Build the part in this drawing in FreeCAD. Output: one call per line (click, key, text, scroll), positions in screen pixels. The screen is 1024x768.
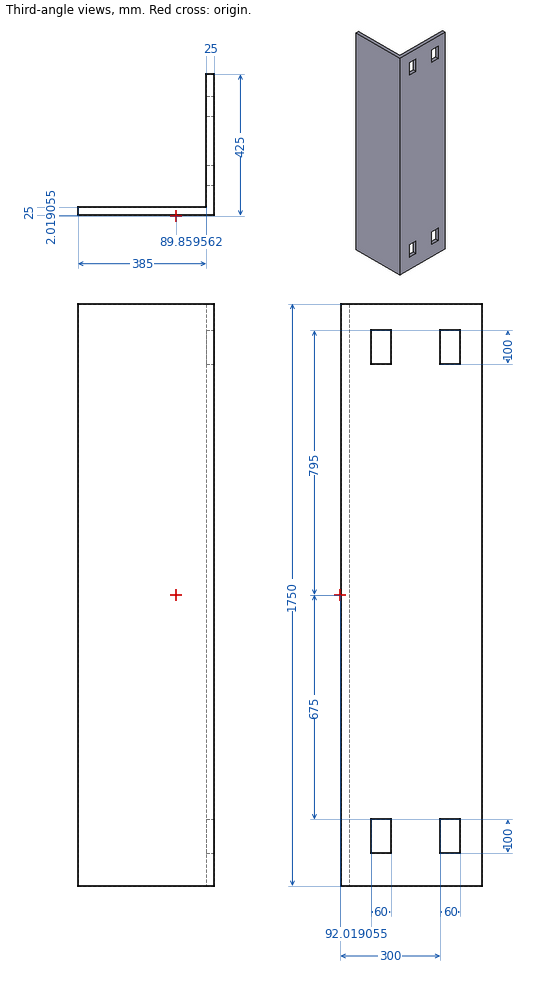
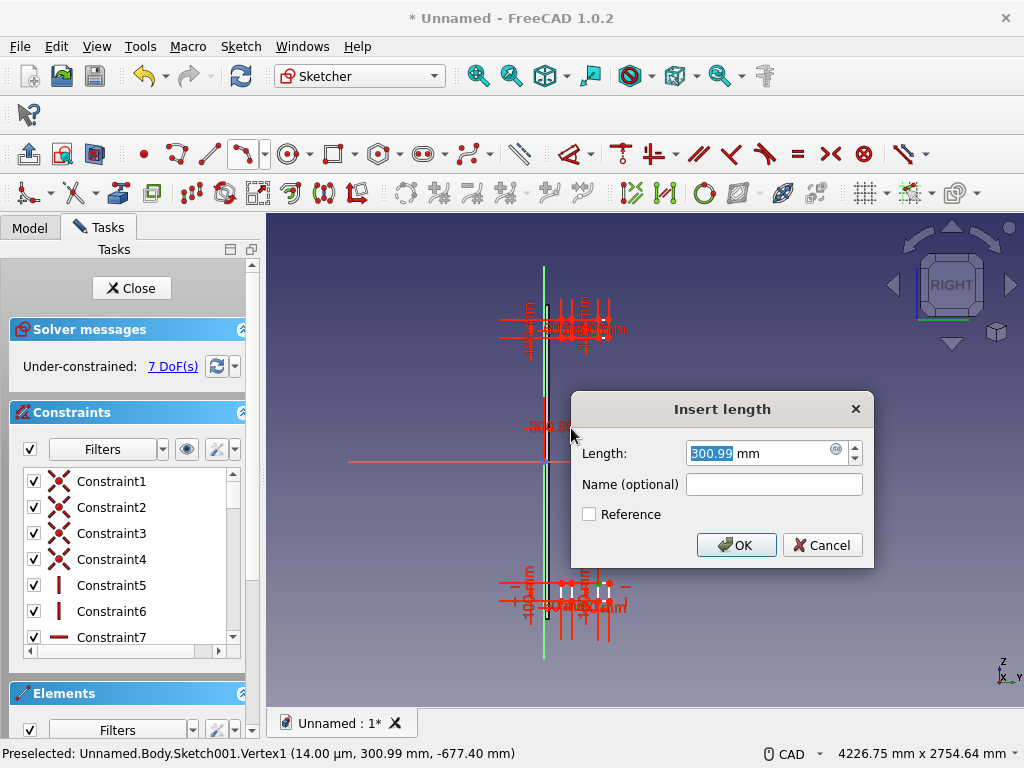
text(300)
key(Return)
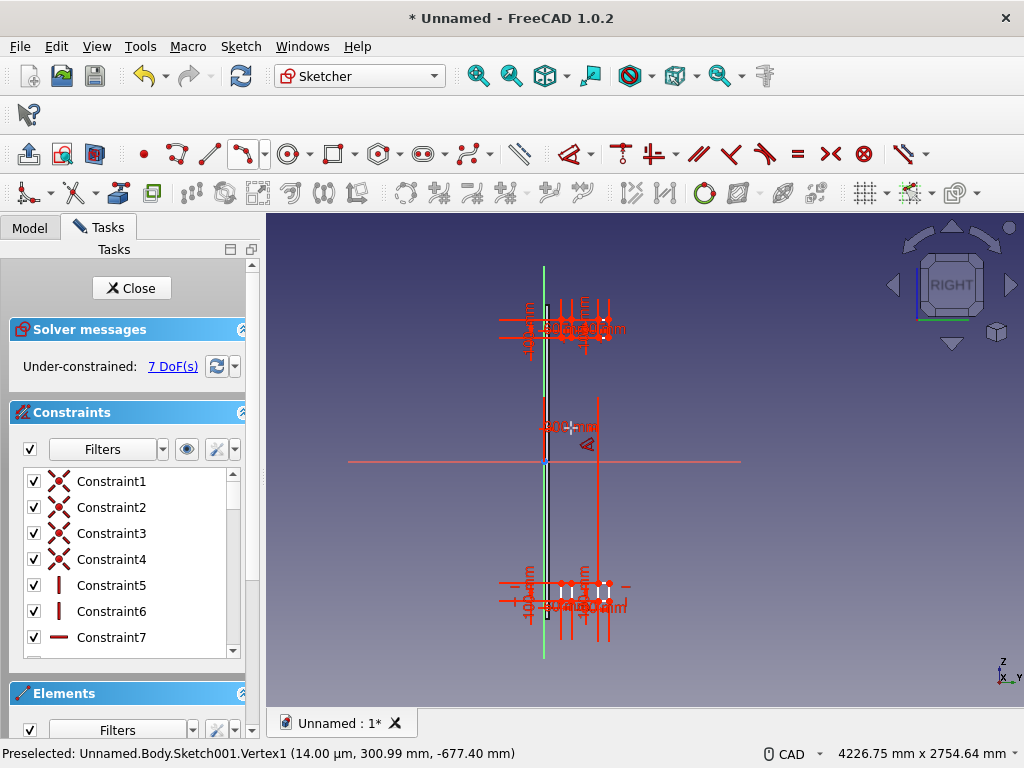
click(598, 583)
click(510, 523)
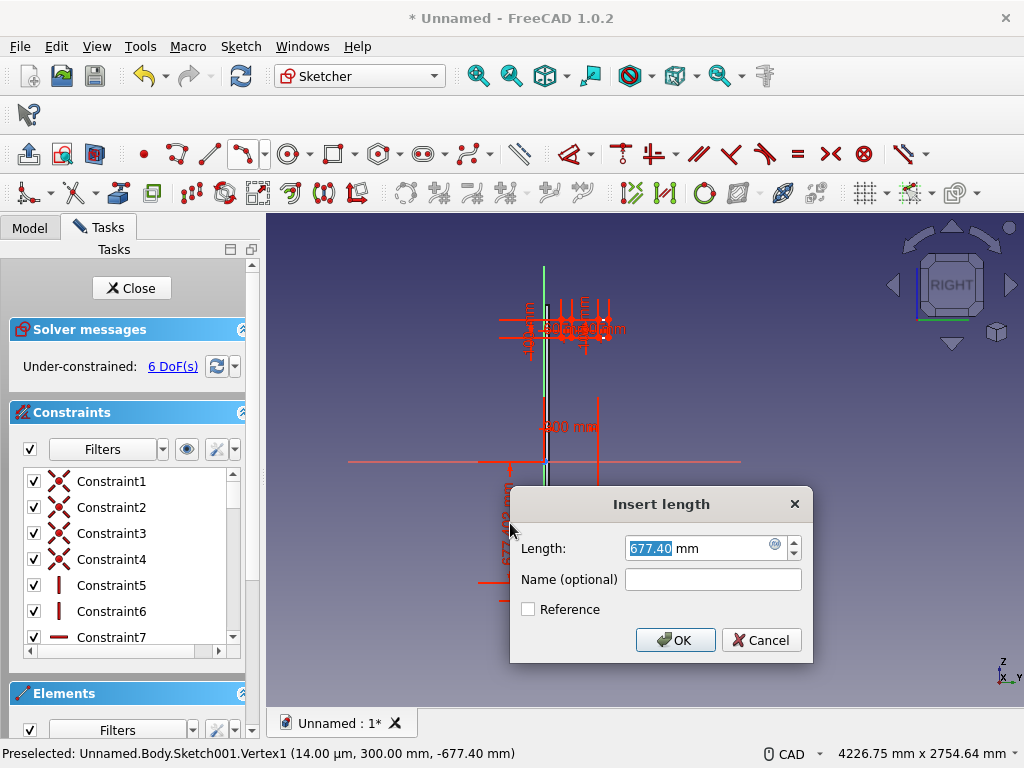
text(675)
key(Return)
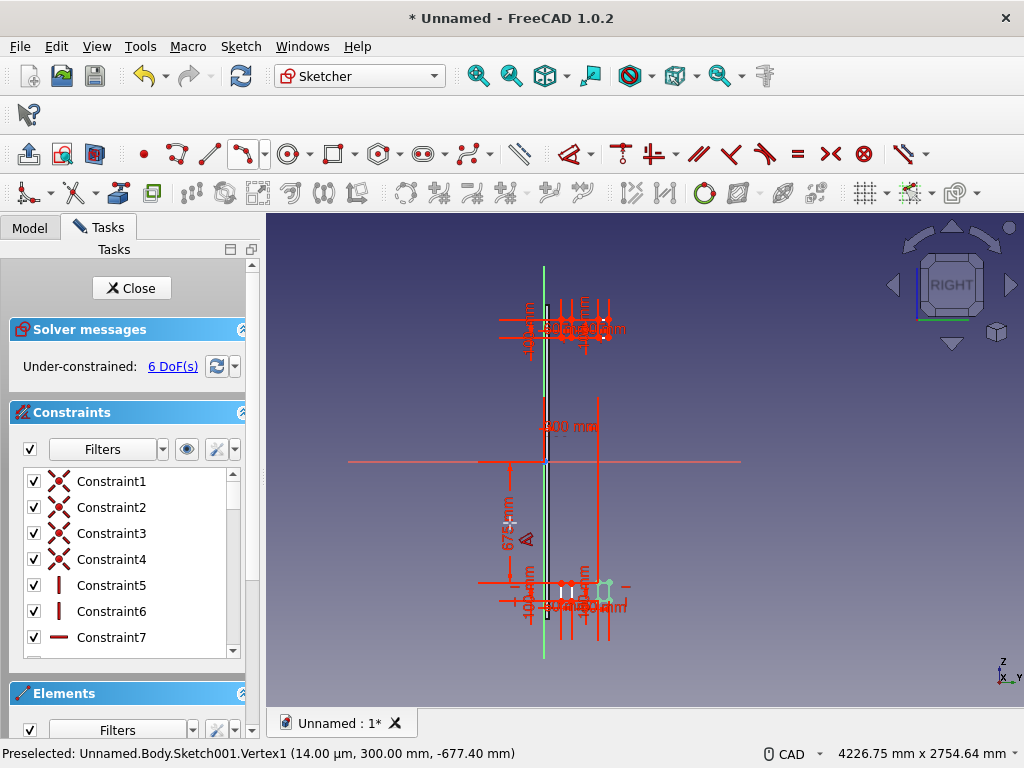
click(598, 320)
click(571, 286)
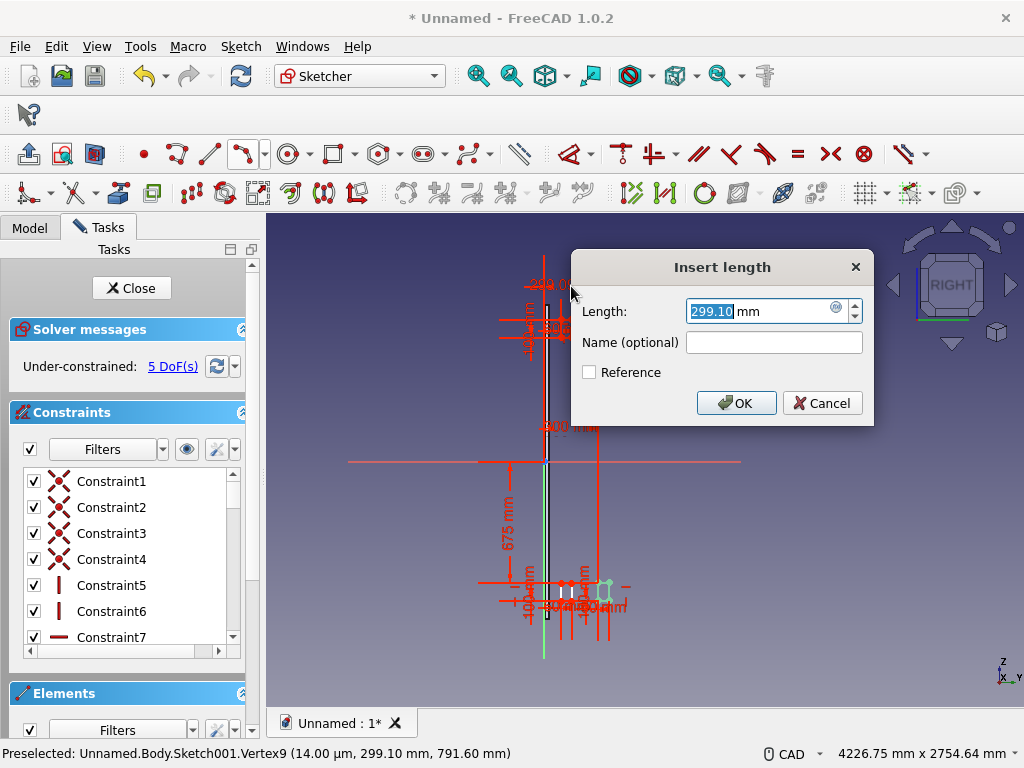
text(300)
key(Return)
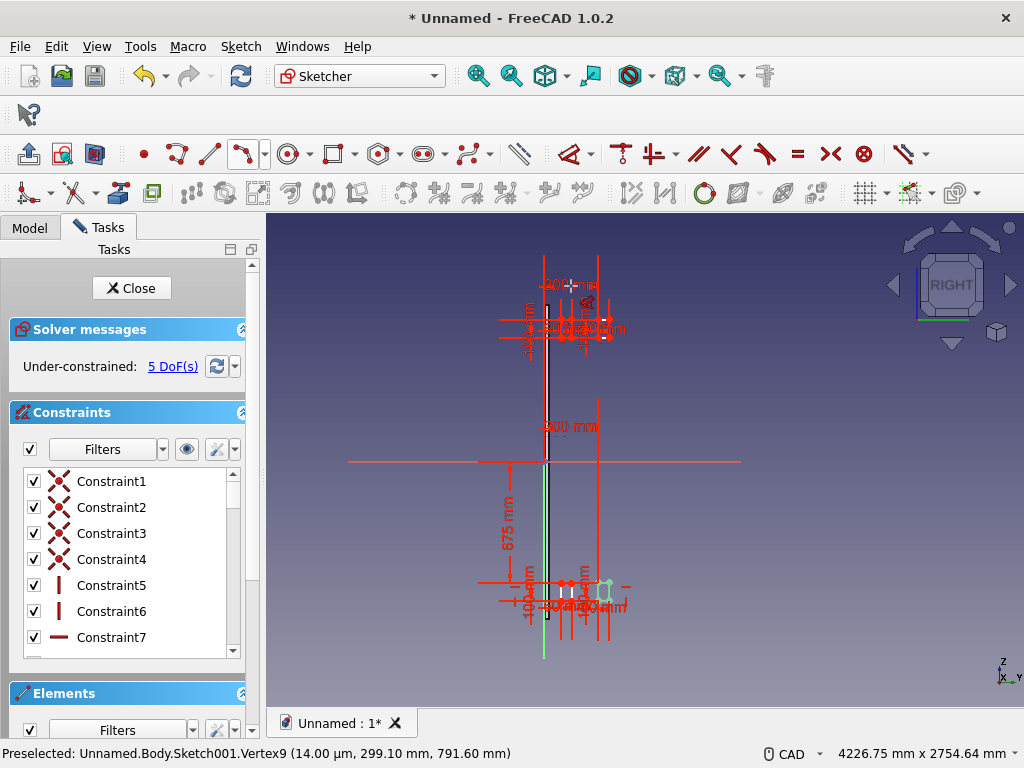
click(598, 320)
click(510, 391)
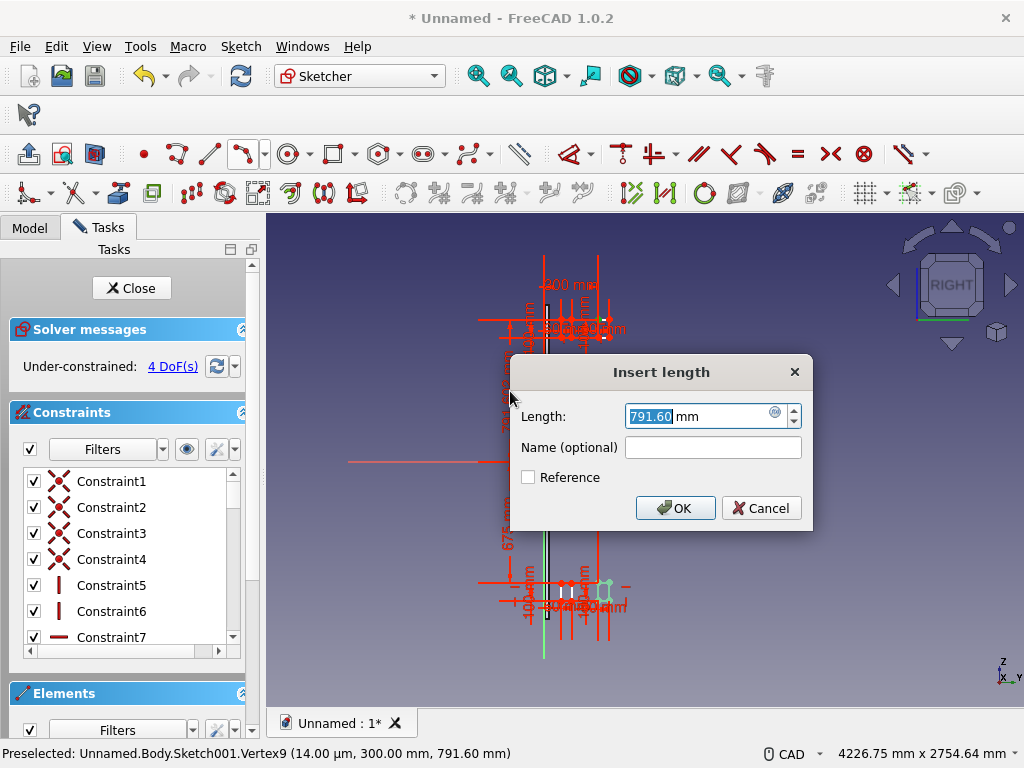
text(795)
key(Return)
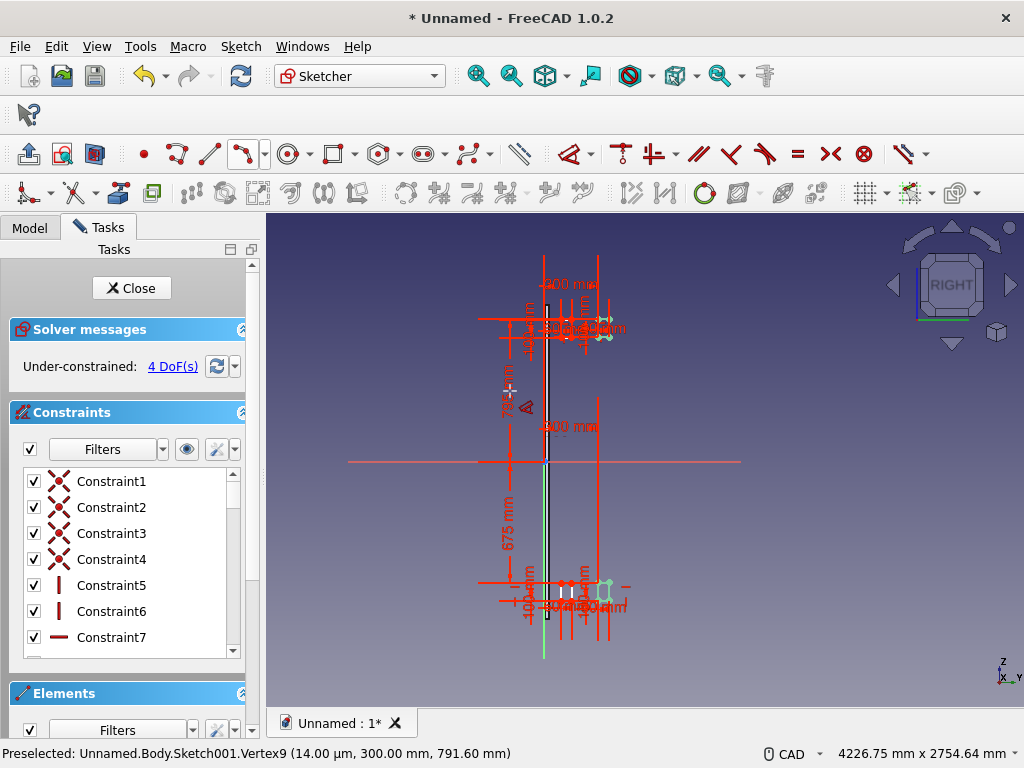
click(561, 583)
click(510, 495)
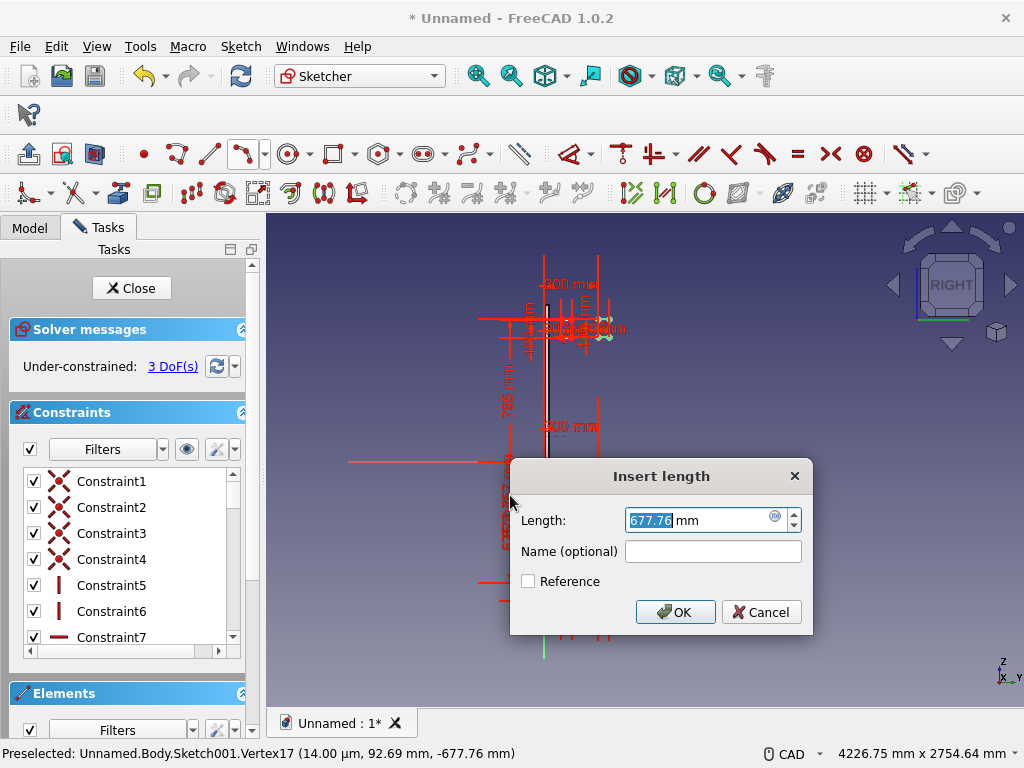
text(675)
key(Return)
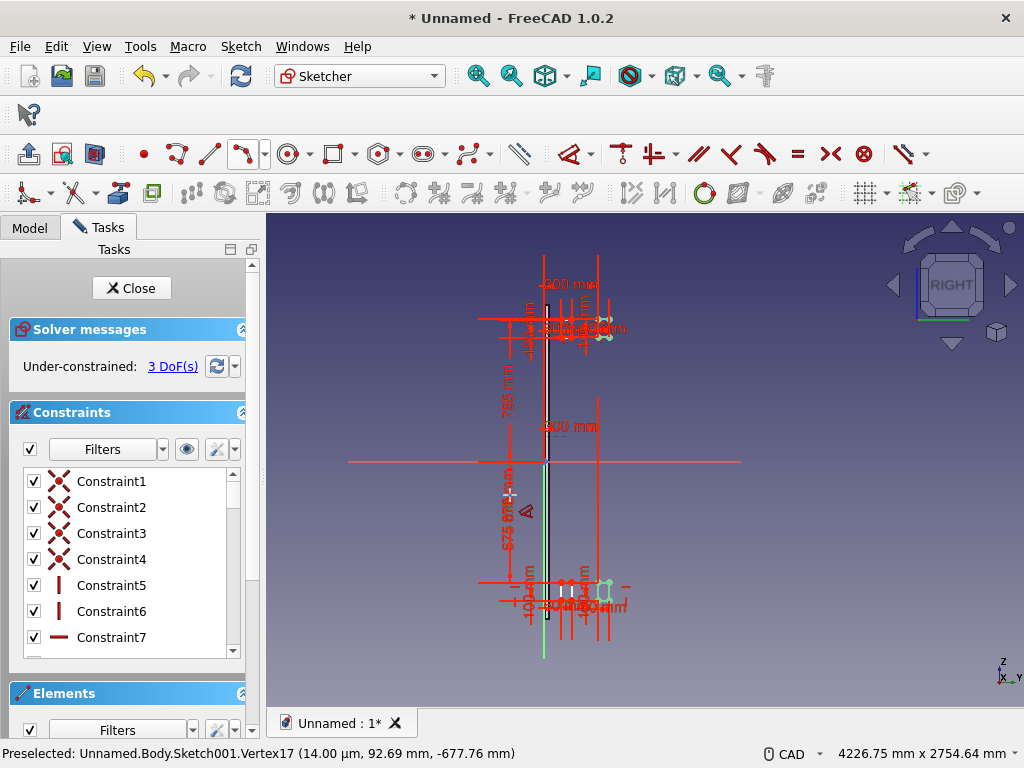
click(561, 320)
click(510, 358)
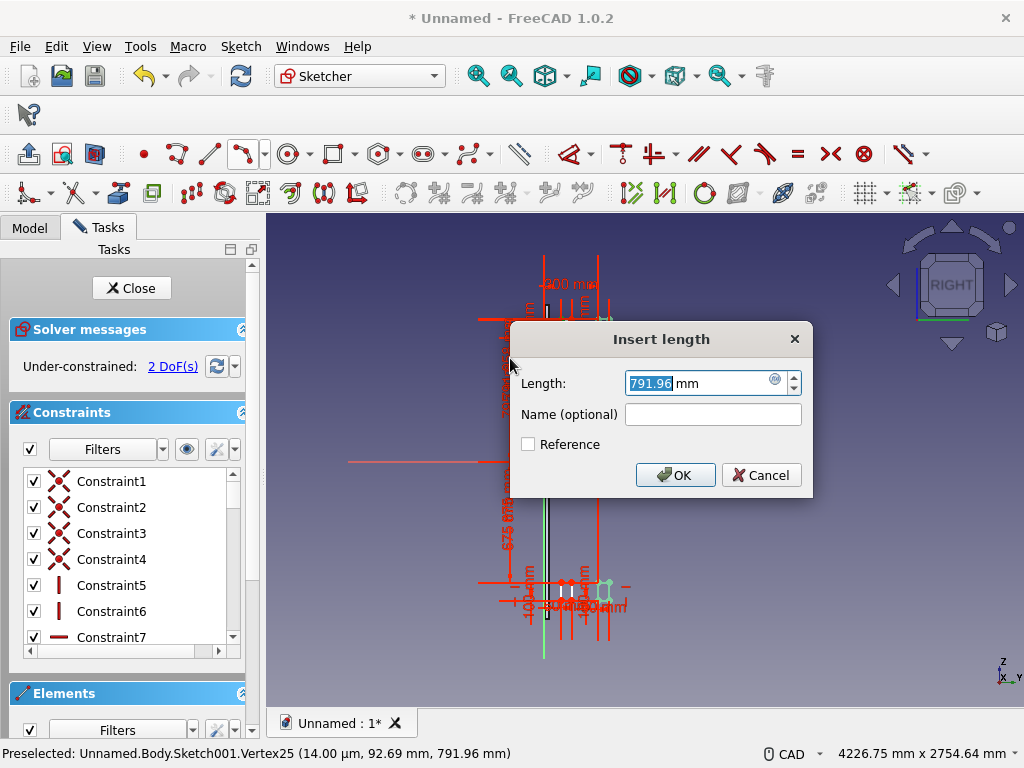
text(795)
key(Return)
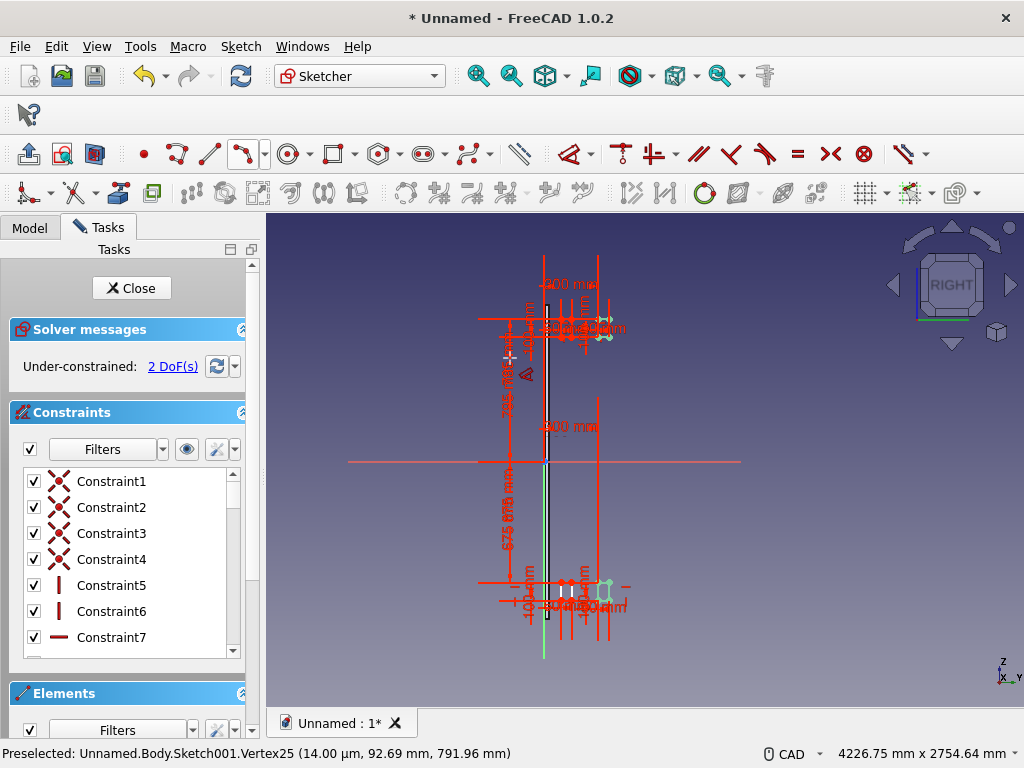
scroll(561, 583, up, 5)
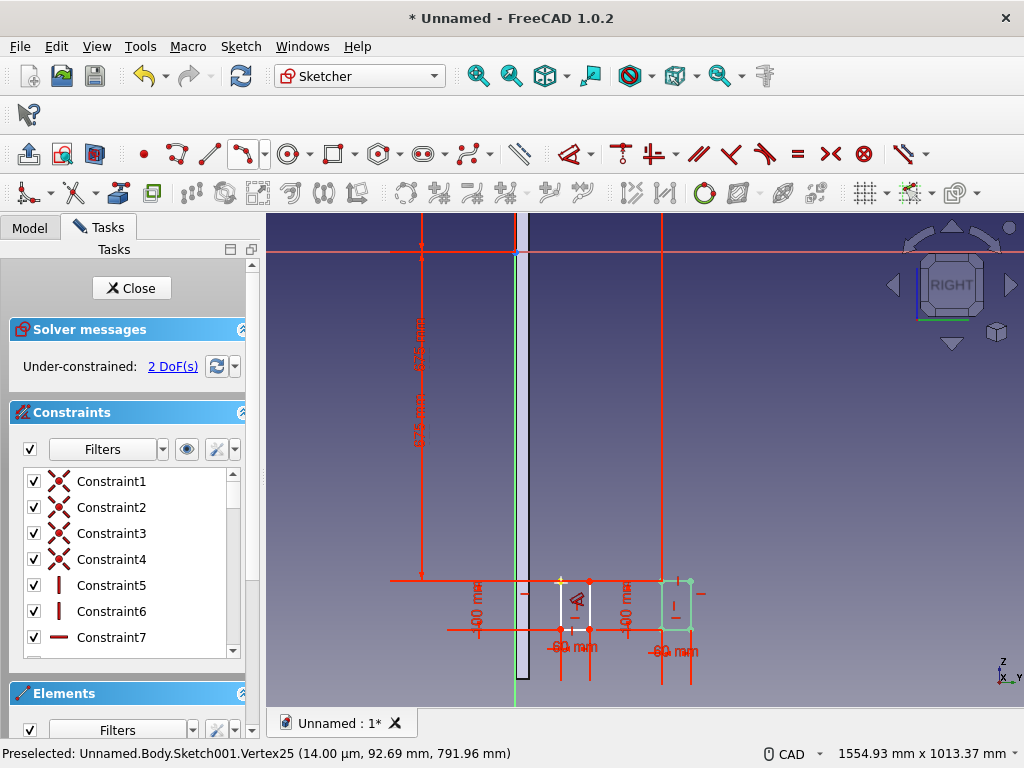
click(561, 581)
click(538, 615)